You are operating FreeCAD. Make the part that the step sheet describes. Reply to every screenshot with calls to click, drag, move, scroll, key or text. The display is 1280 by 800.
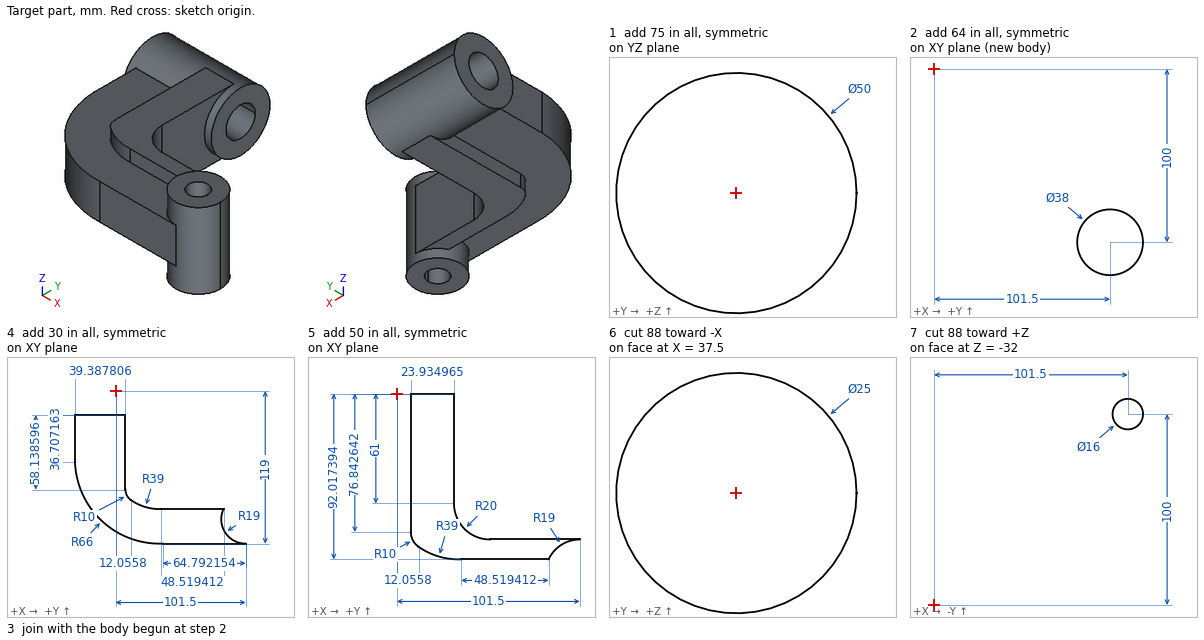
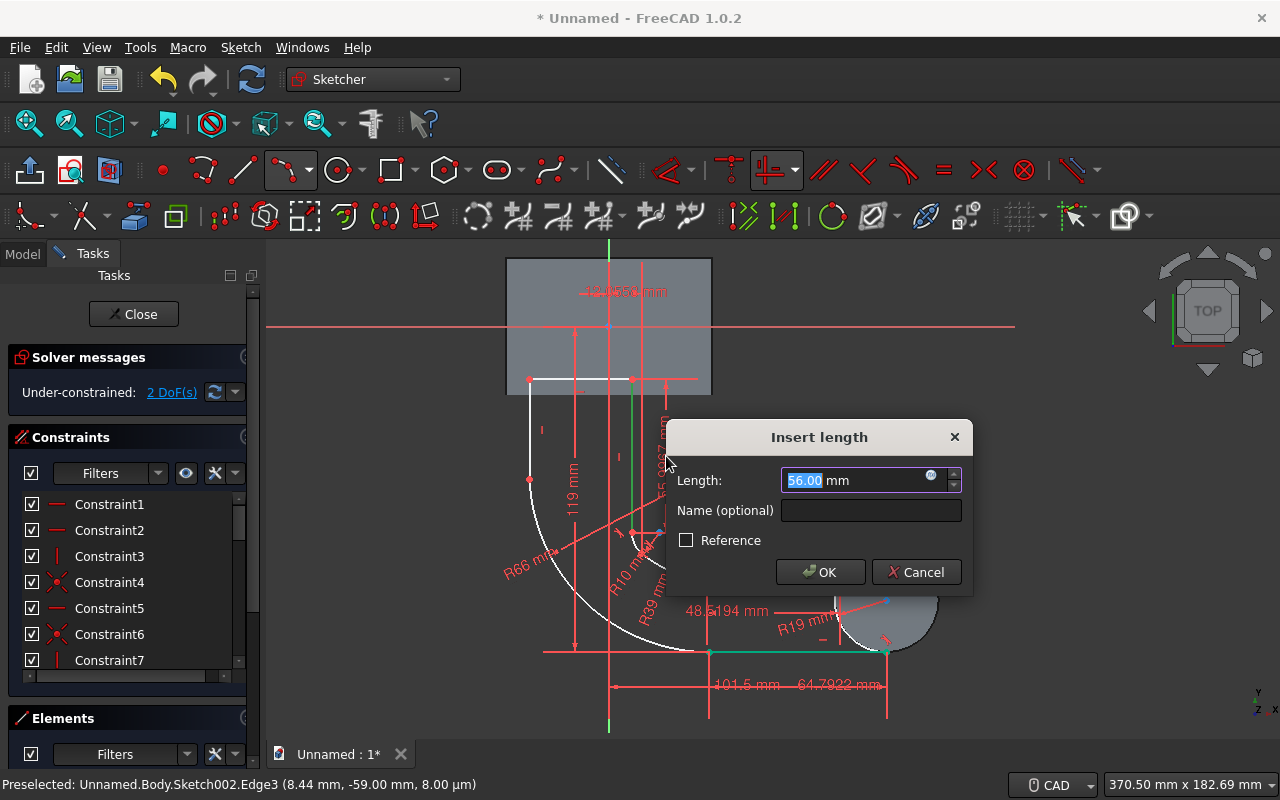
text(58.138596)
key(Return)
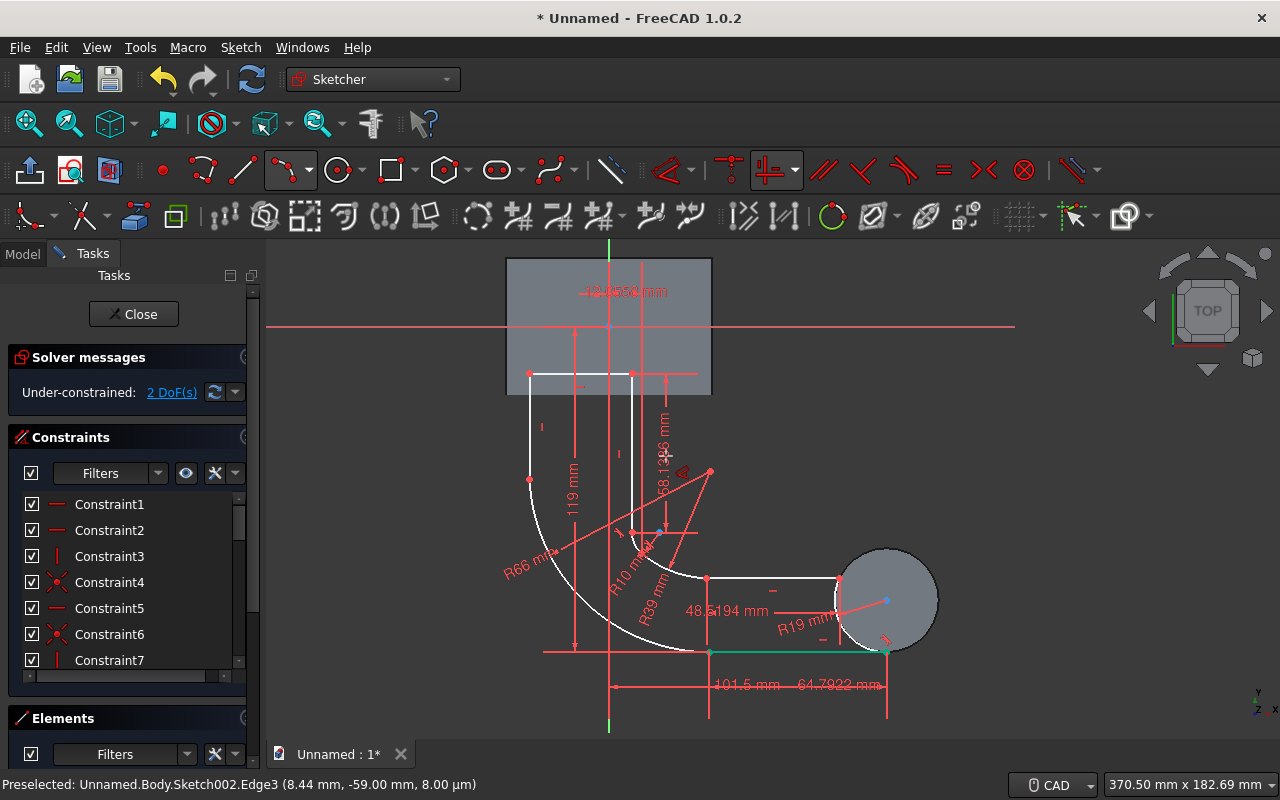
click(560, 374)
click(581, 340)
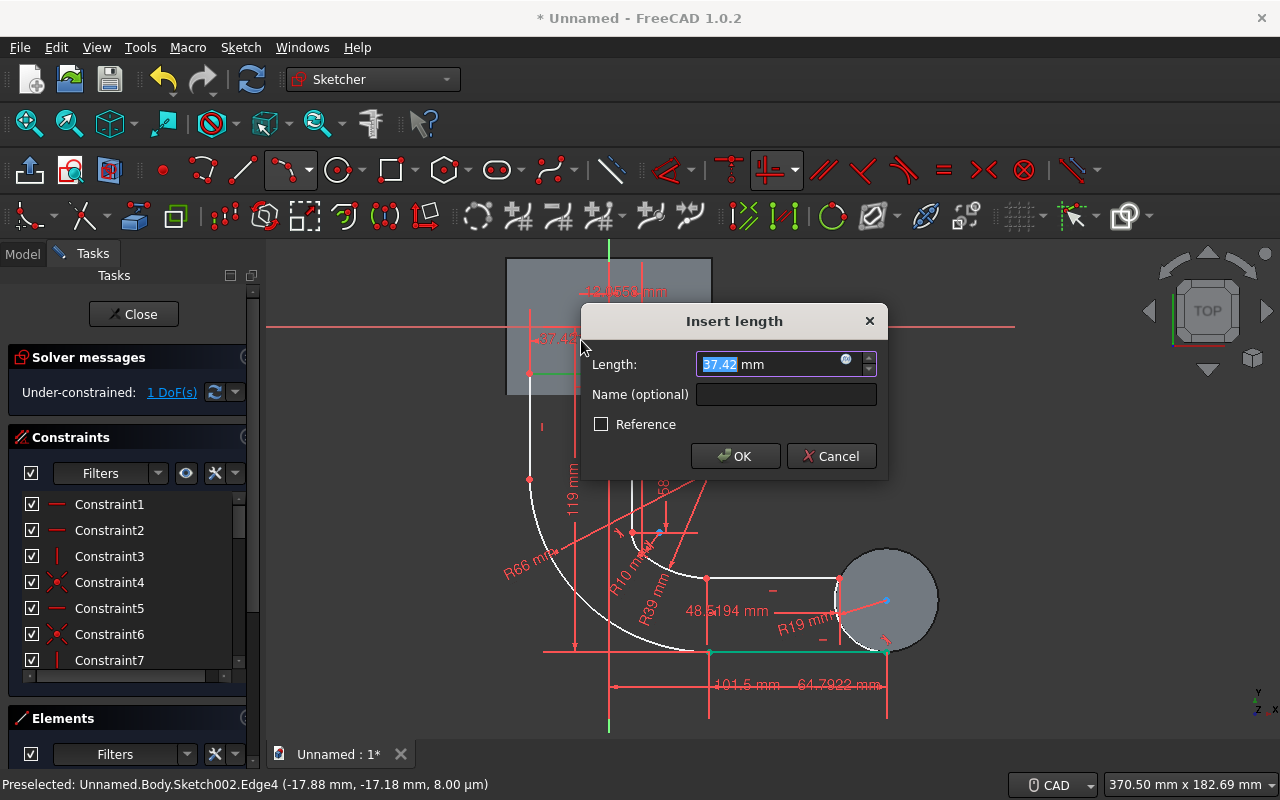
text(39.387806)
key(Return)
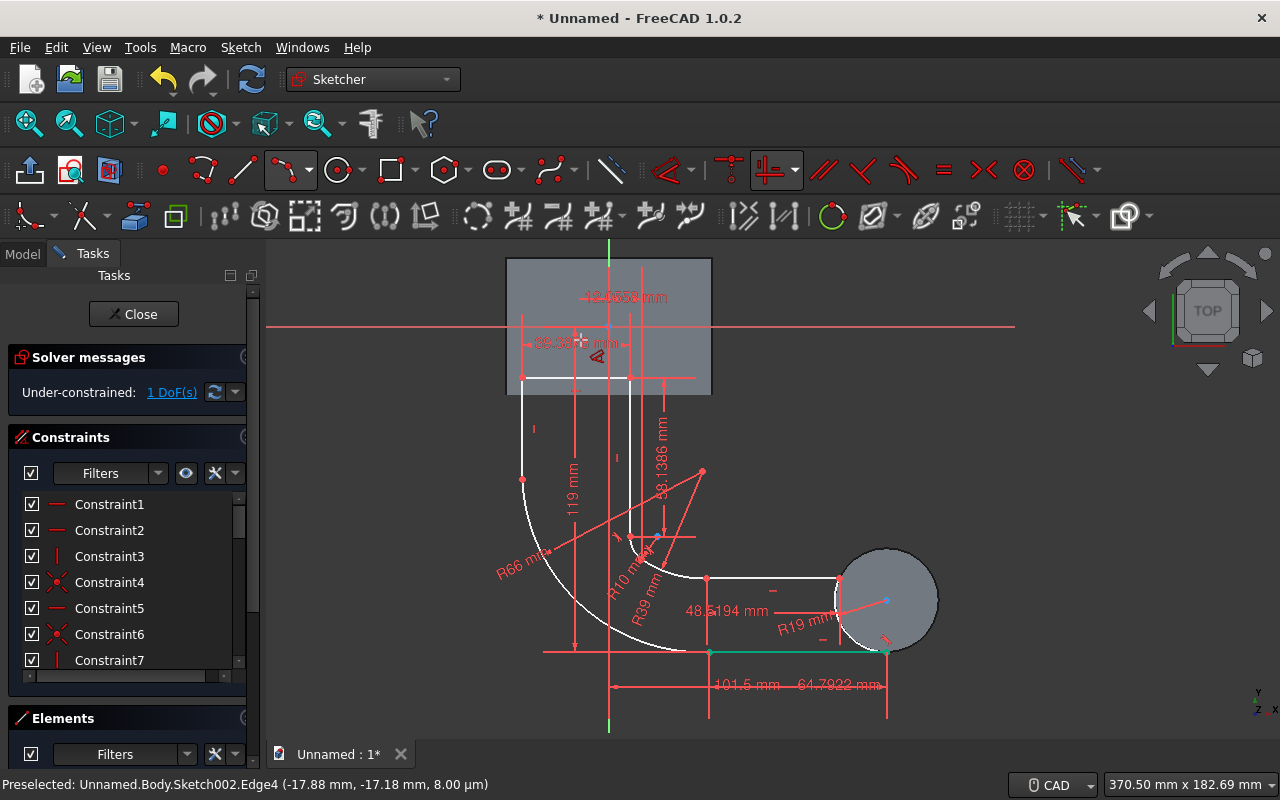
click(522, 408)
click(488, 429)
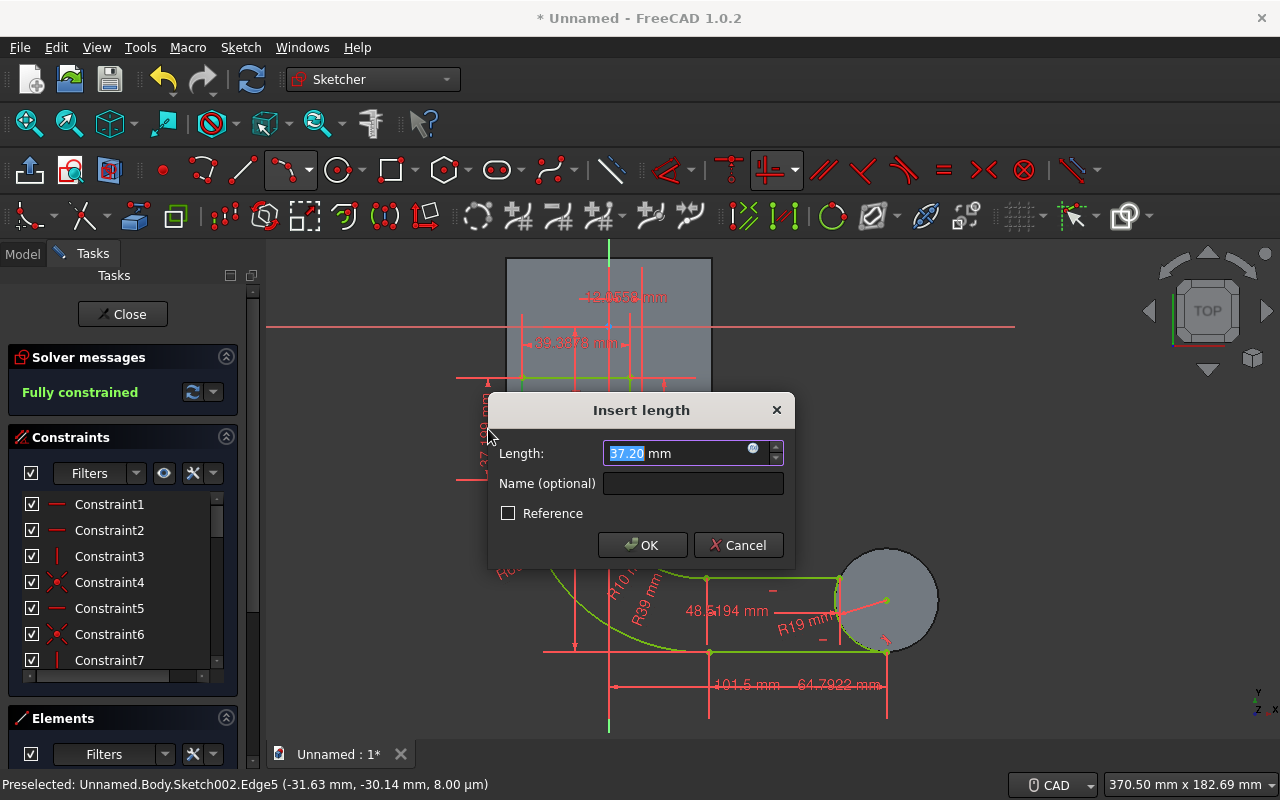
text(36.707163)
key(Return)
key(Escape)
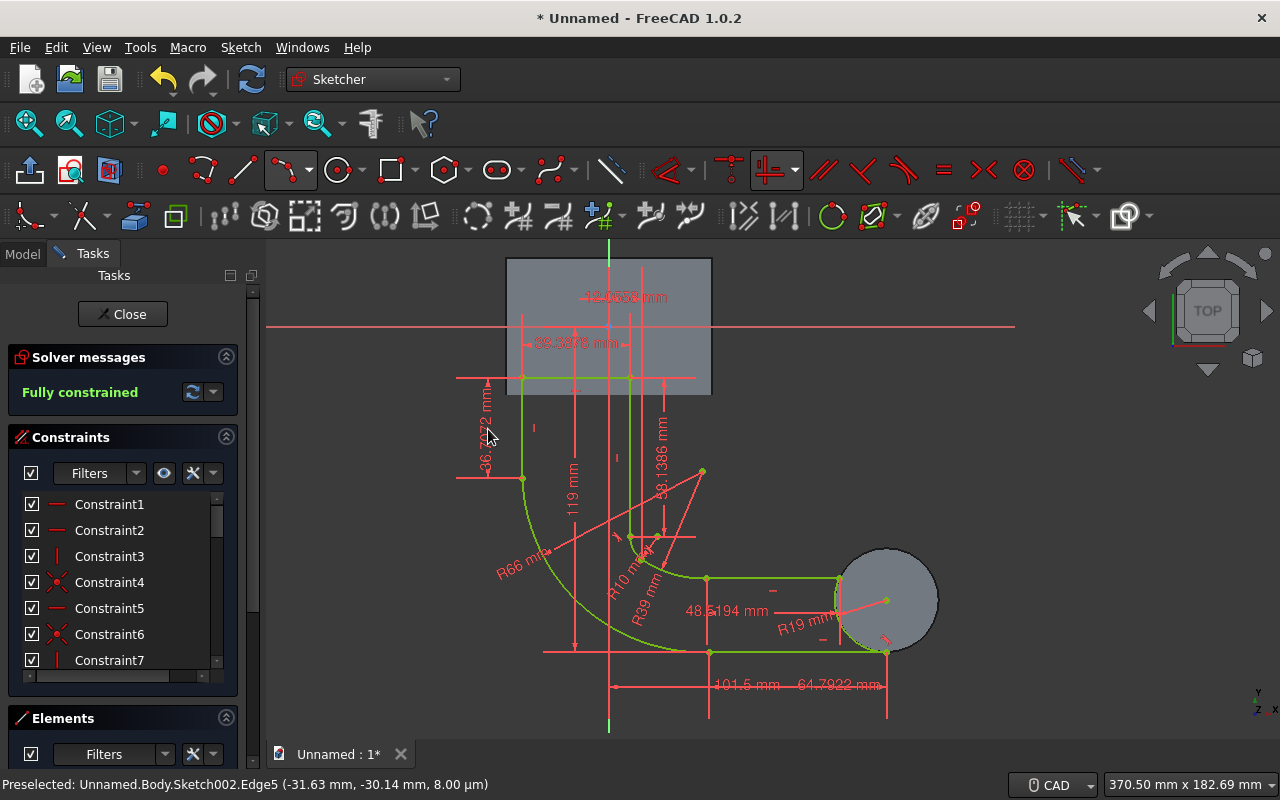
click(123, 314)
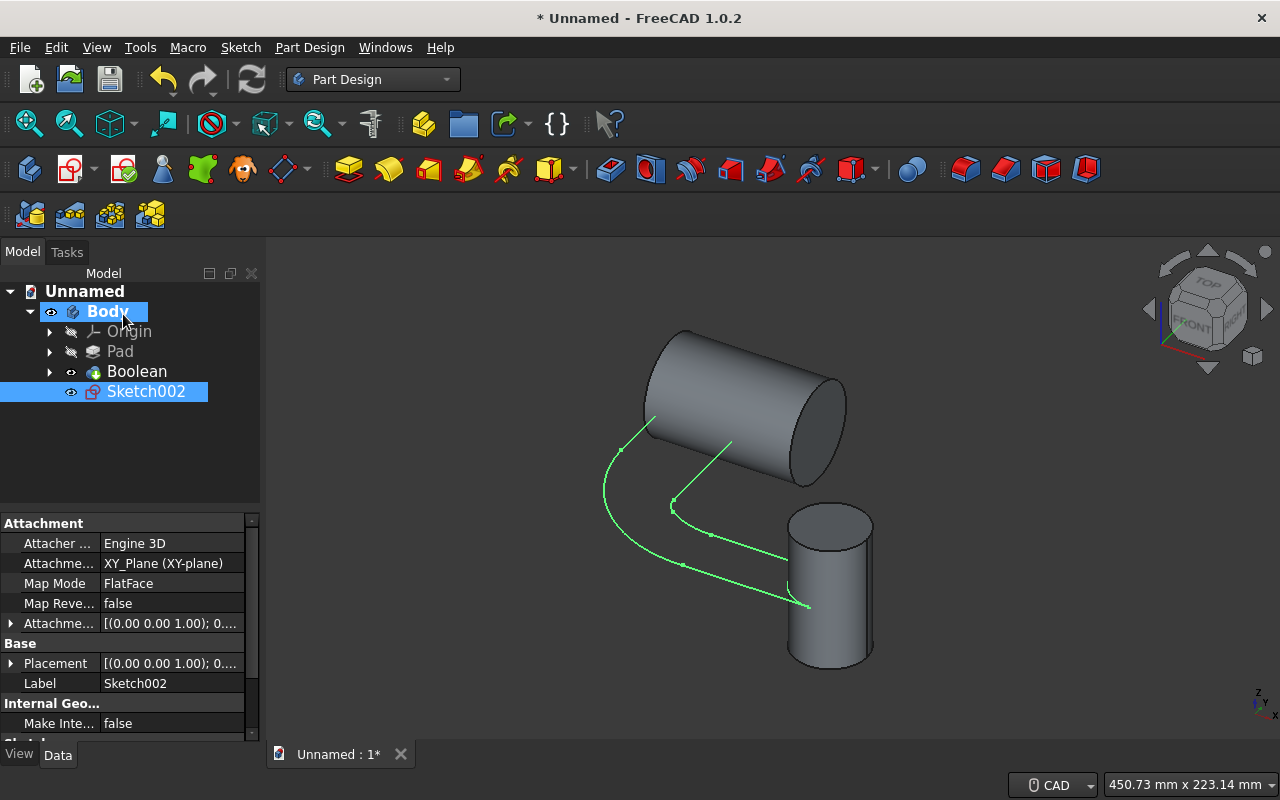
click(350, 170)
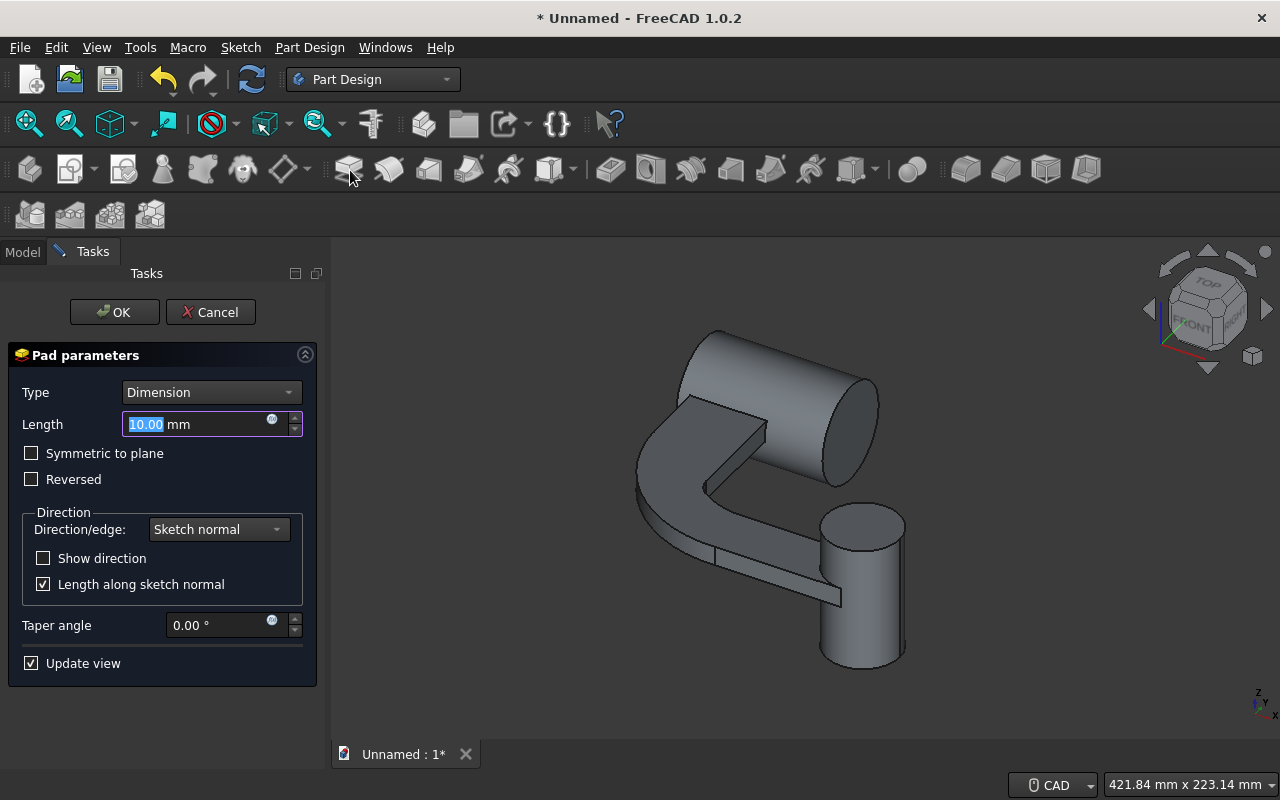
text(30)
key(Tab)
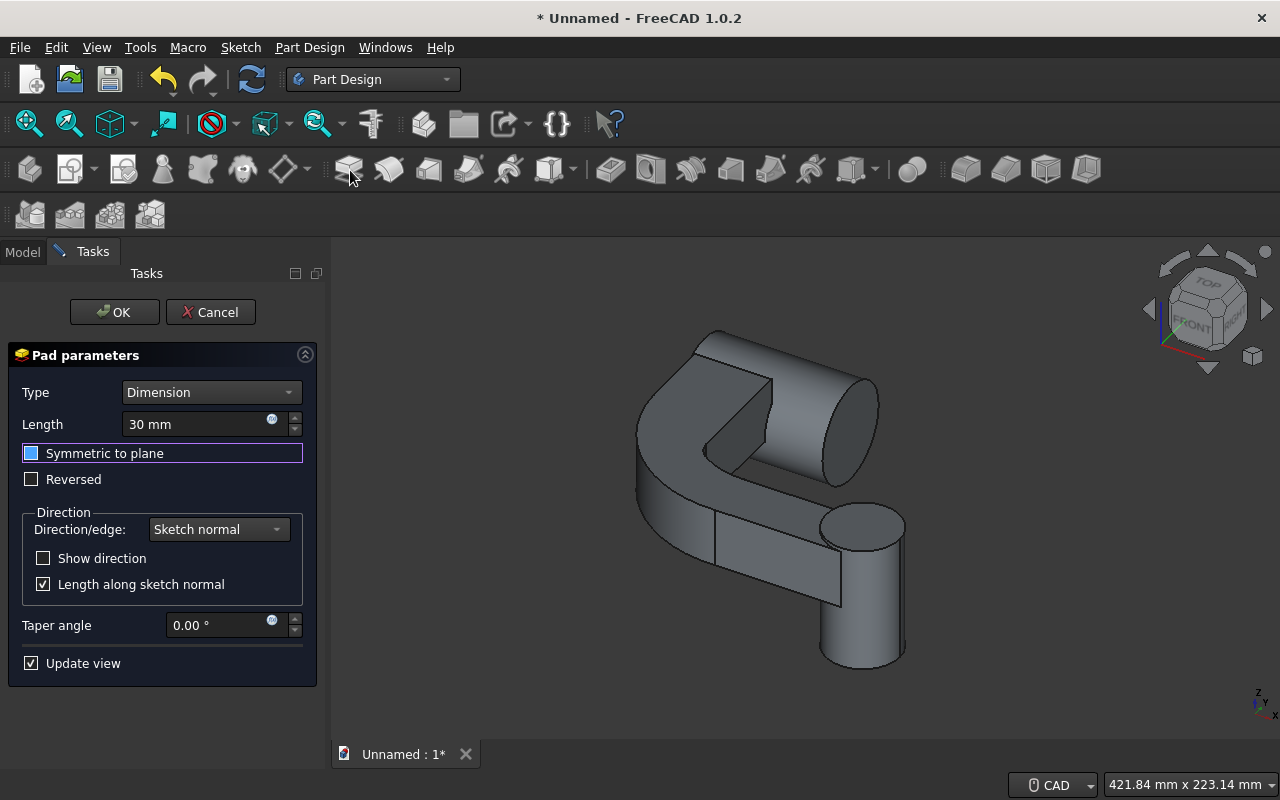
click(30, 453)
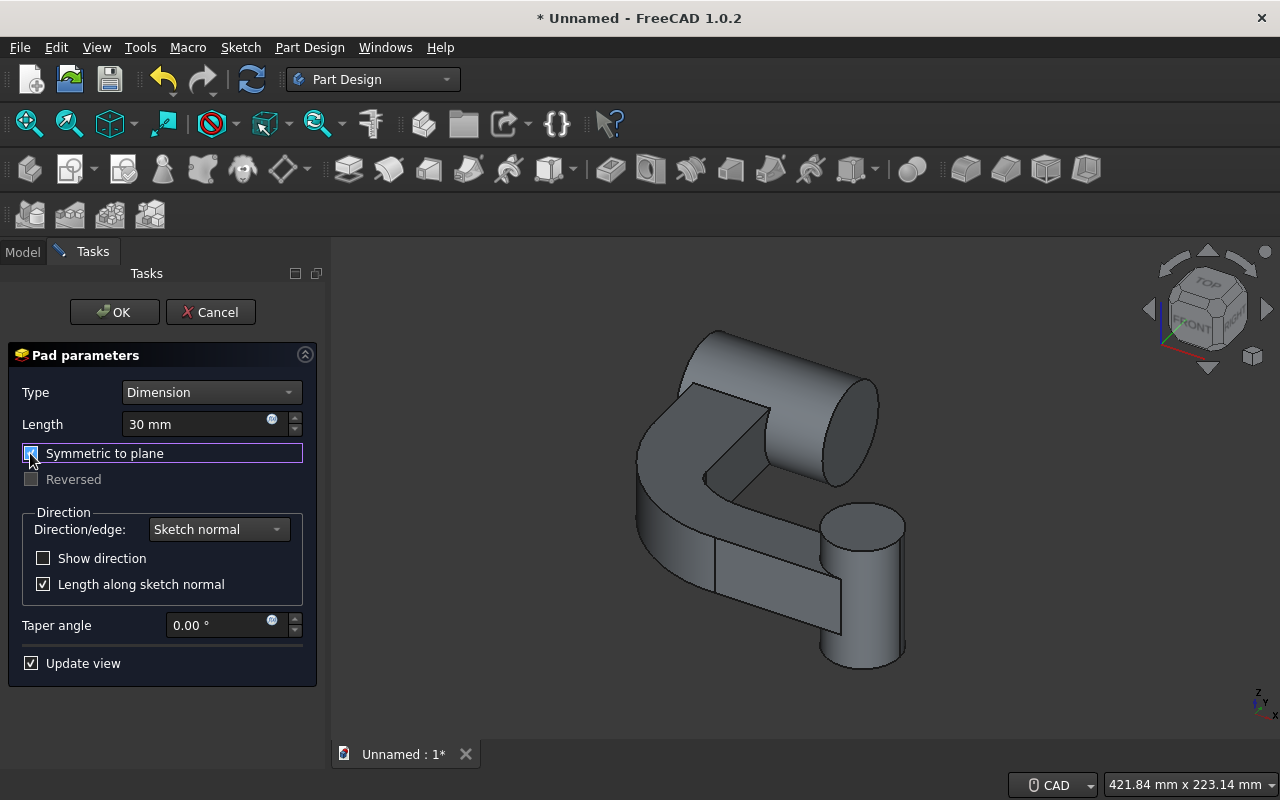
click(115, 312)